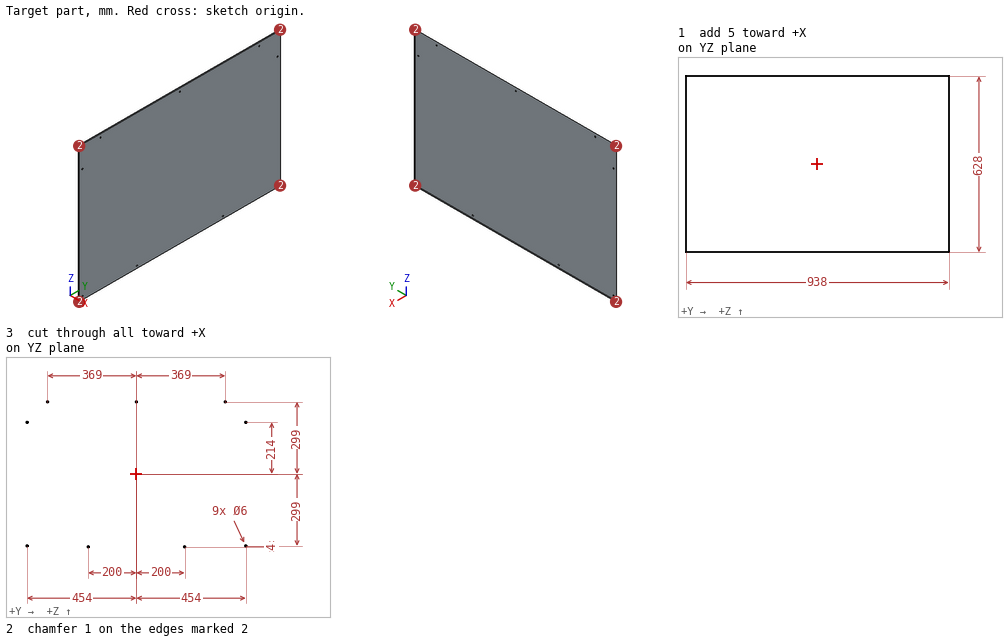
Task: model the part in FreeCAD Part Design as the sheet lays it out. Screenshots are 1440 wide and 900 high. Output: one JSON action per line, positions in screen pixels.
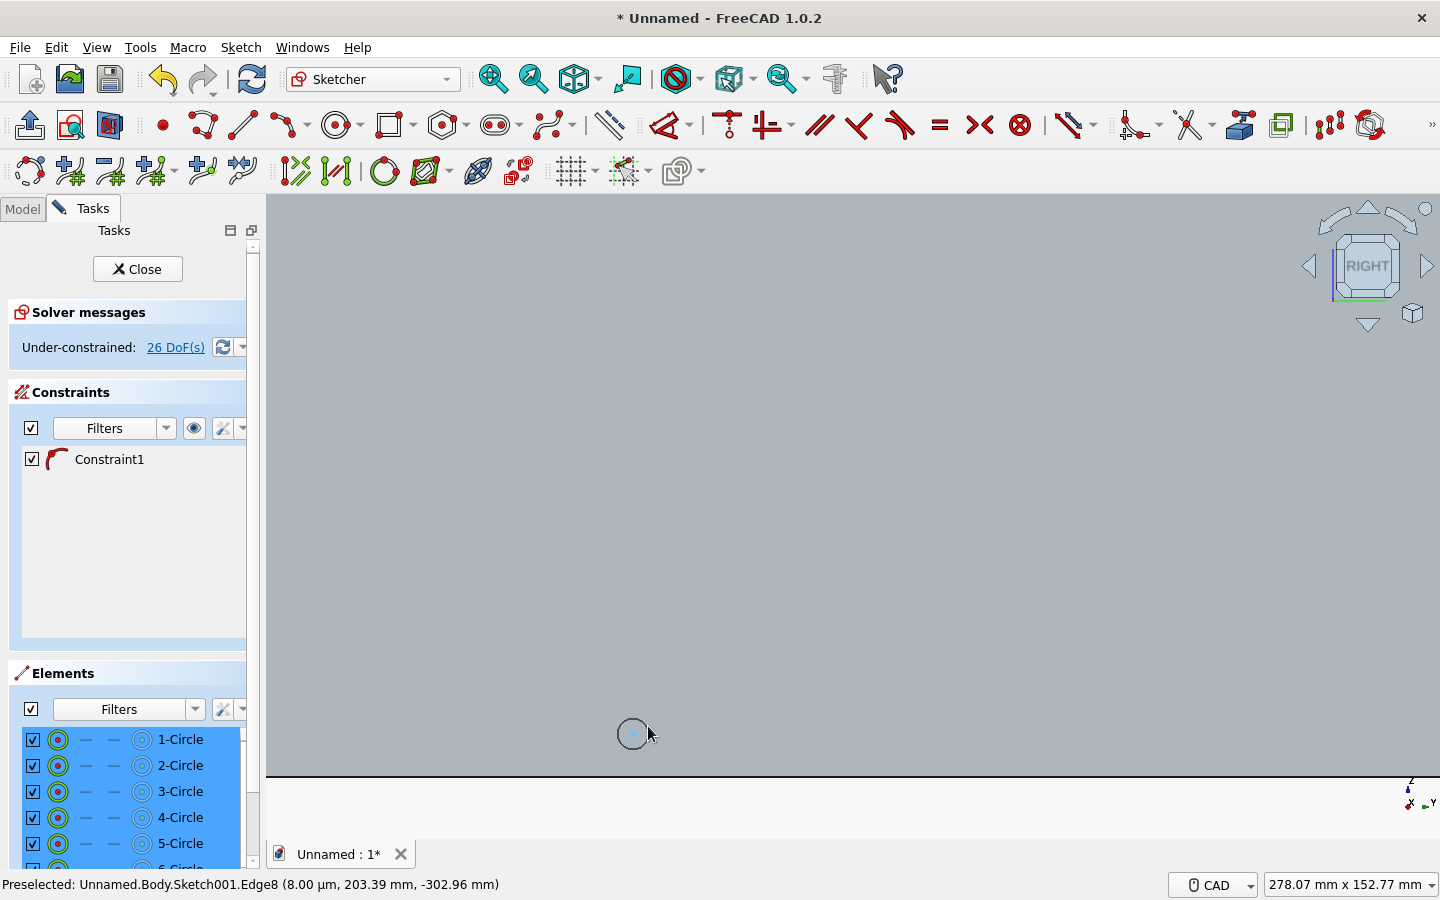
{"action": "left_click", "coordinate": [644, 723]}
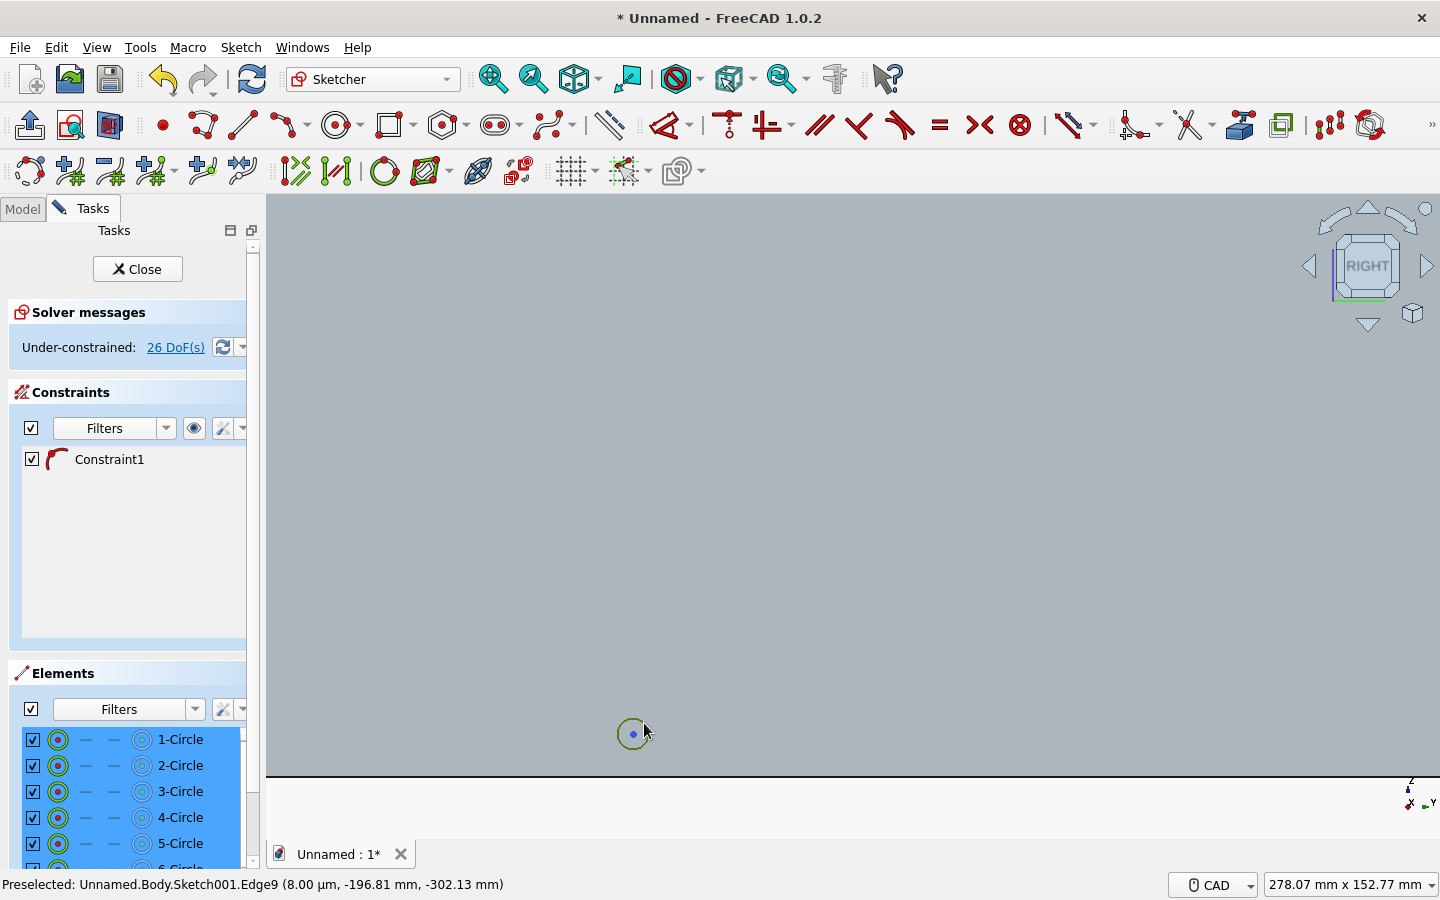
{"action": "left_click", "coordinate": [940, 126]}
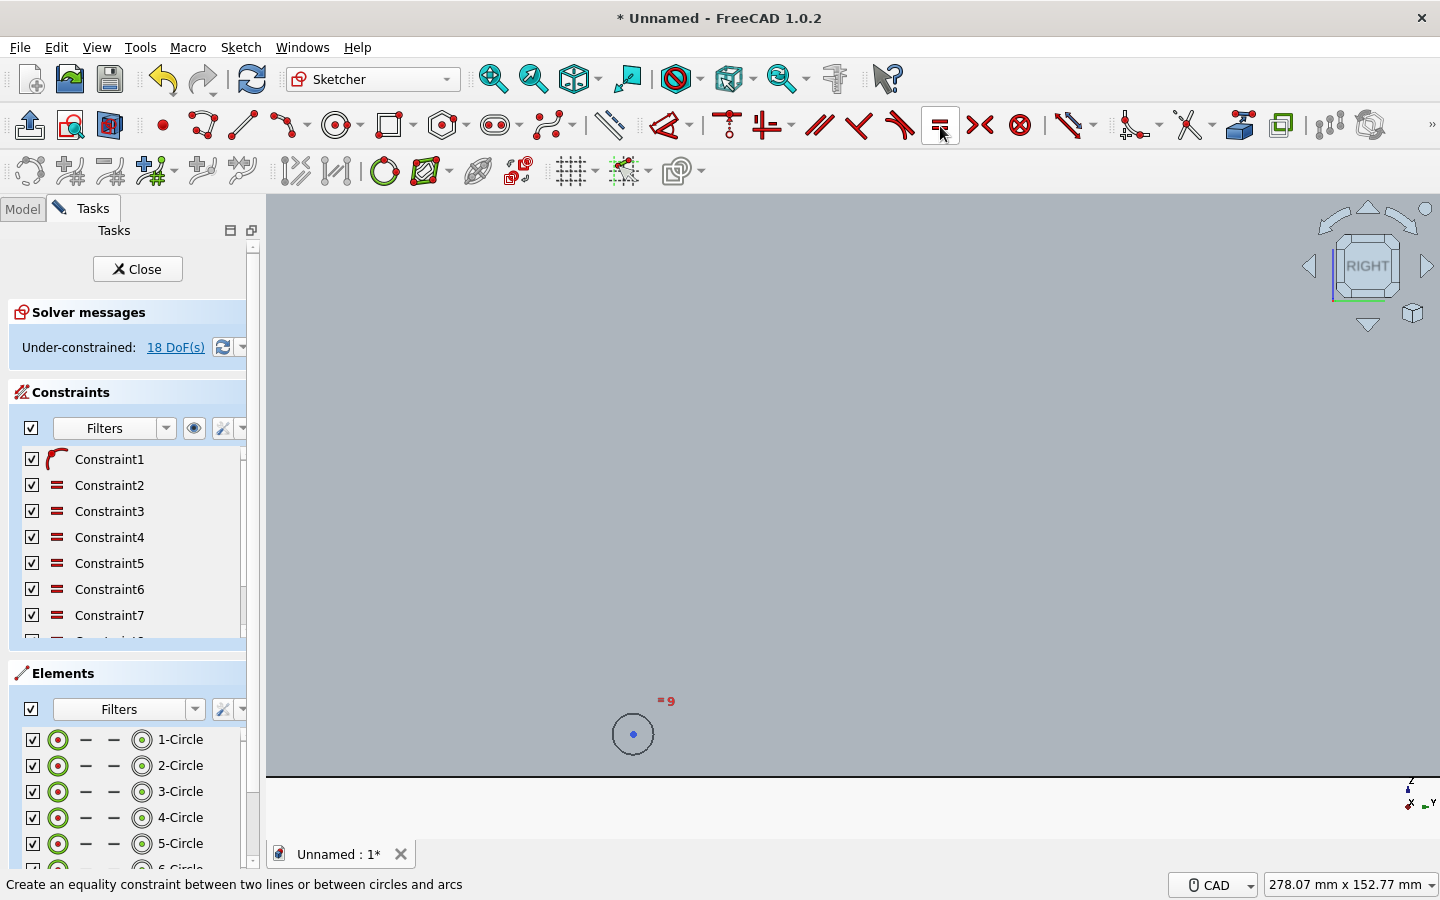
{"action": "scroll", "coordinate": [647, 726], "scroll_direction": "down", "scroll_amount": 9}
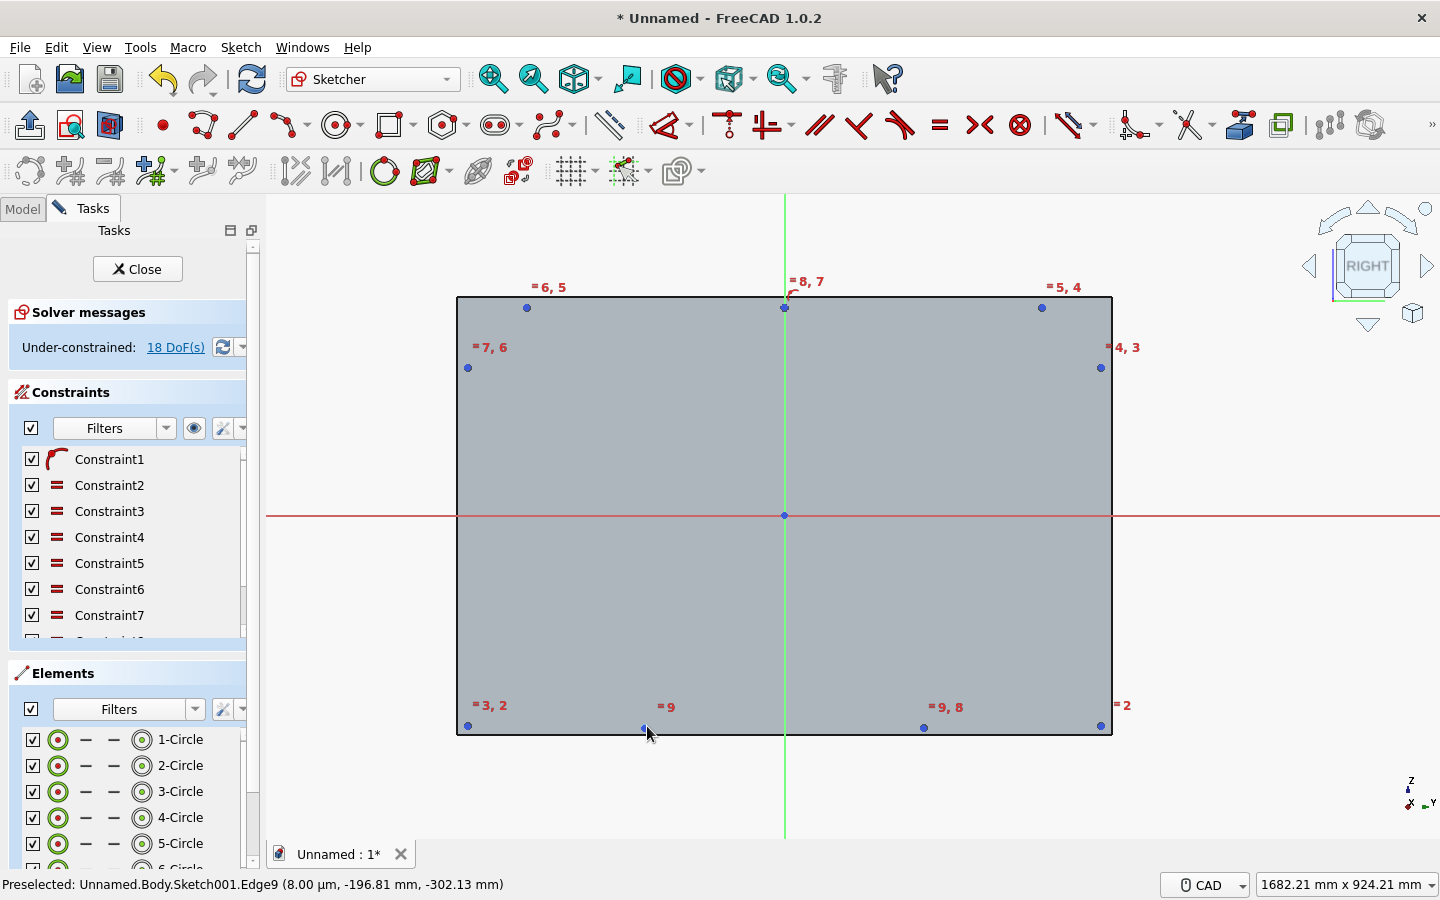
{"action": "left_click", "coordinate": [1101, 726]}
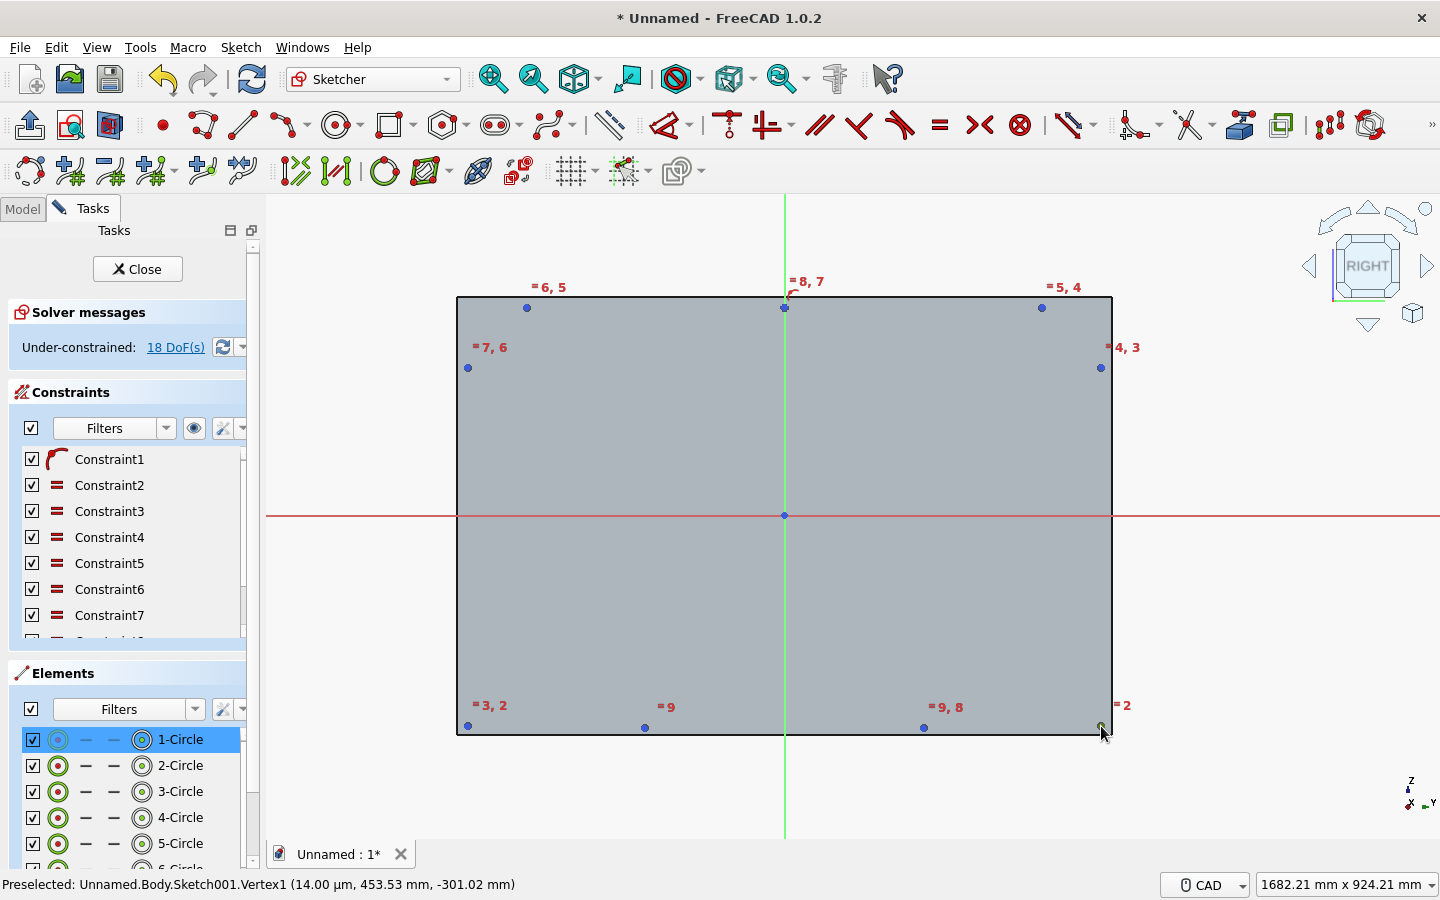
{"action": "left_click", "coordinate": [468, 726]}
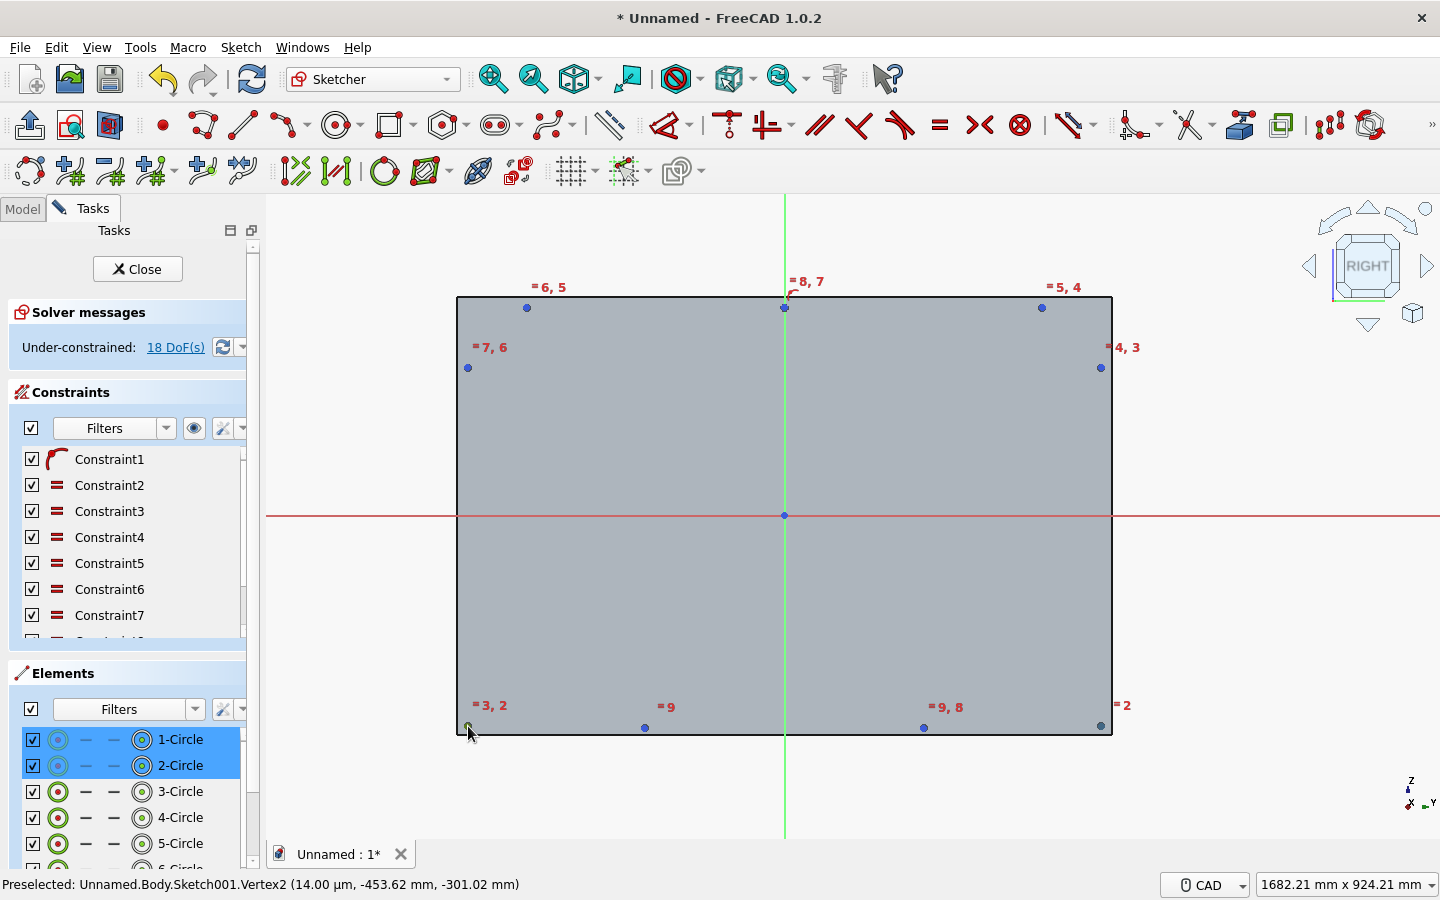
{"action": "key", "text": "h"}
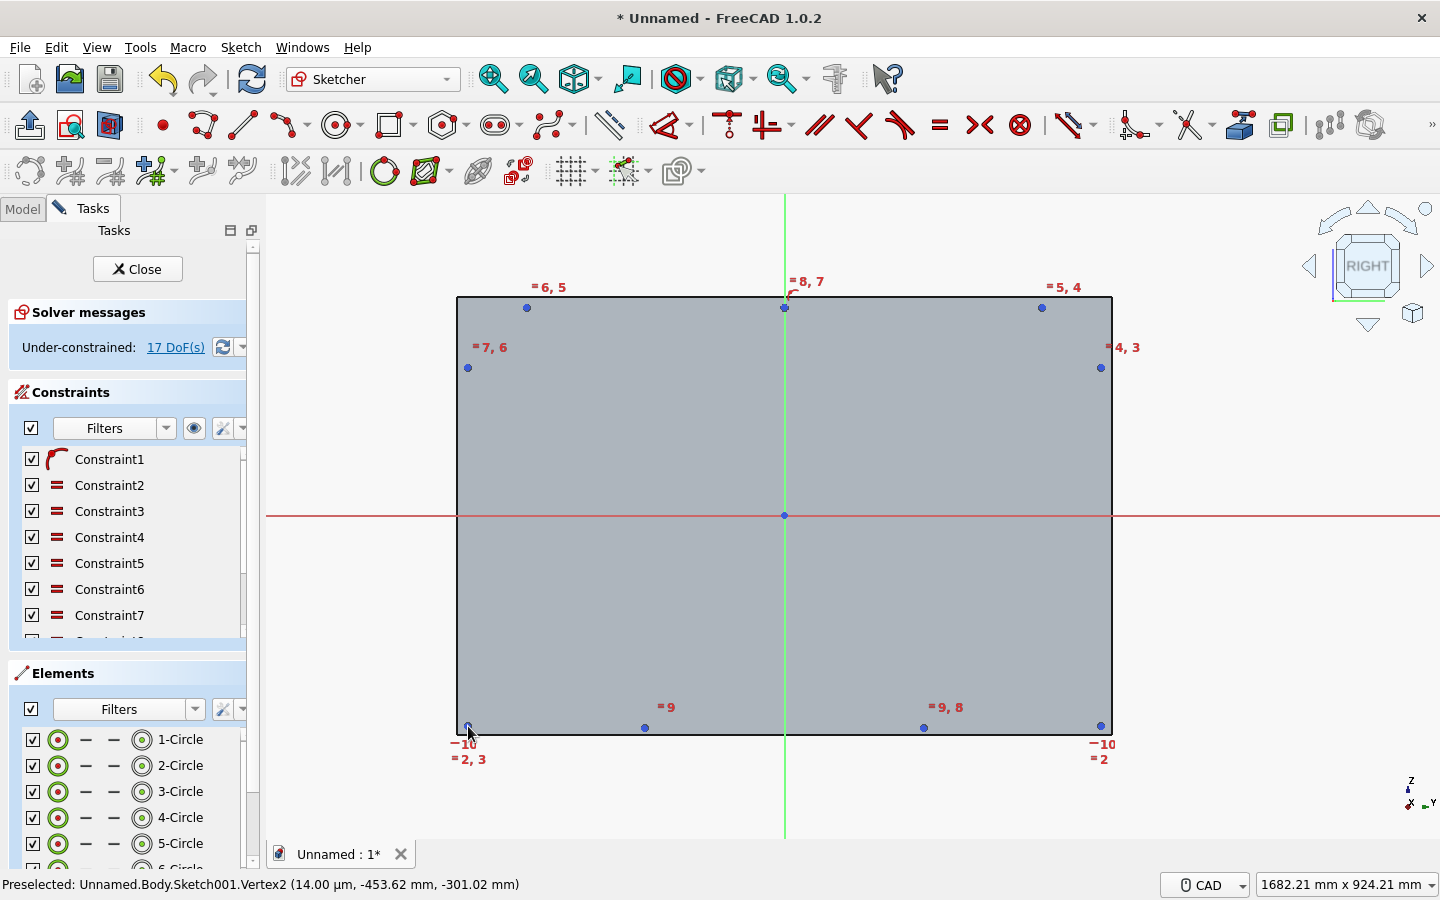
{"action": "left_click", "coordinate": [1101, 726]}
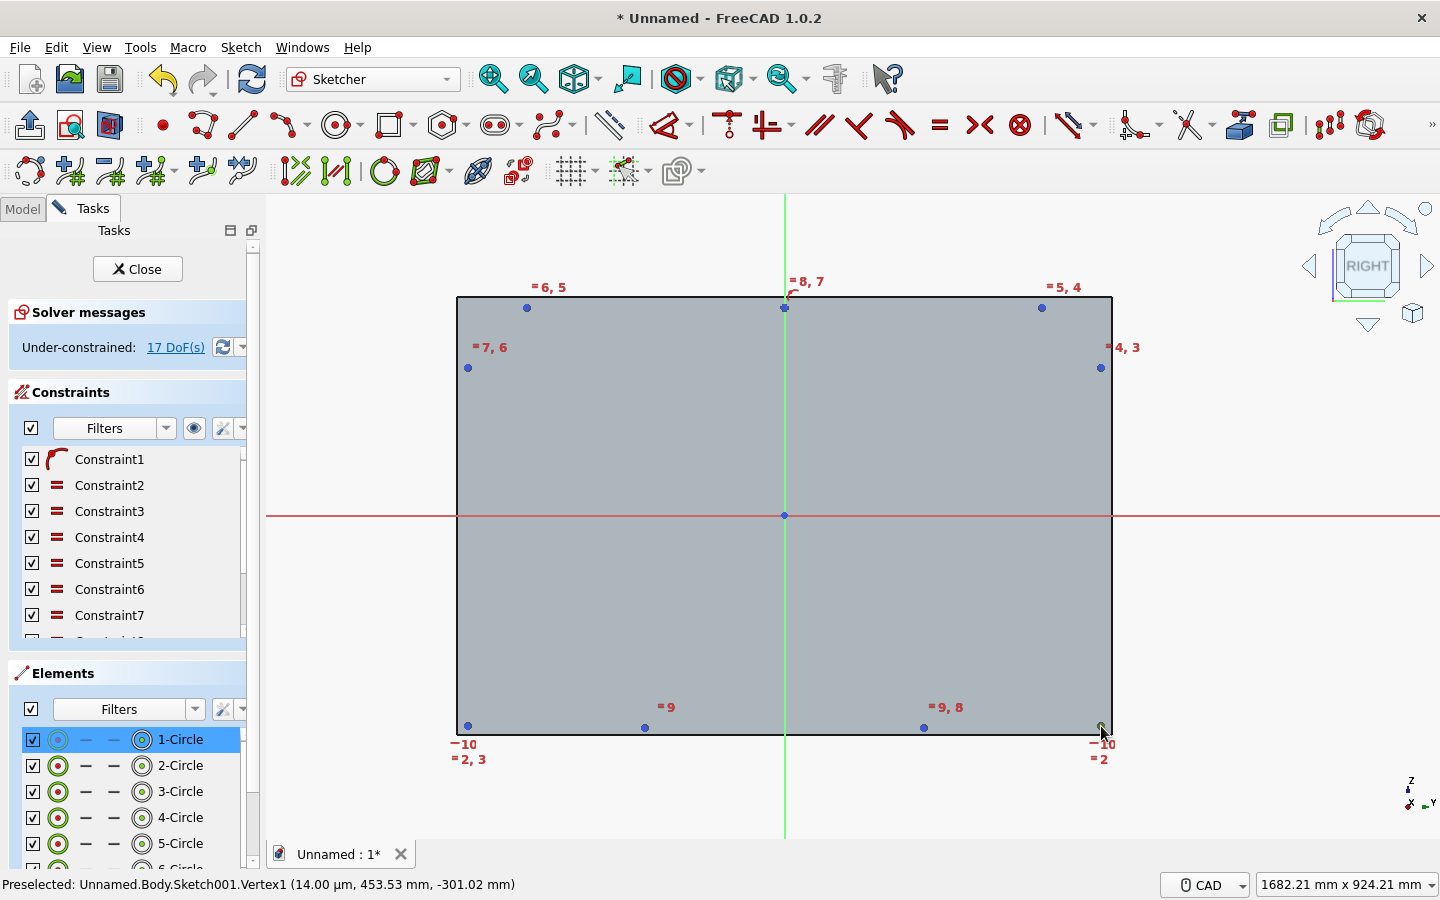
{"action": "left_click", "coordinate": [1101, 368]}